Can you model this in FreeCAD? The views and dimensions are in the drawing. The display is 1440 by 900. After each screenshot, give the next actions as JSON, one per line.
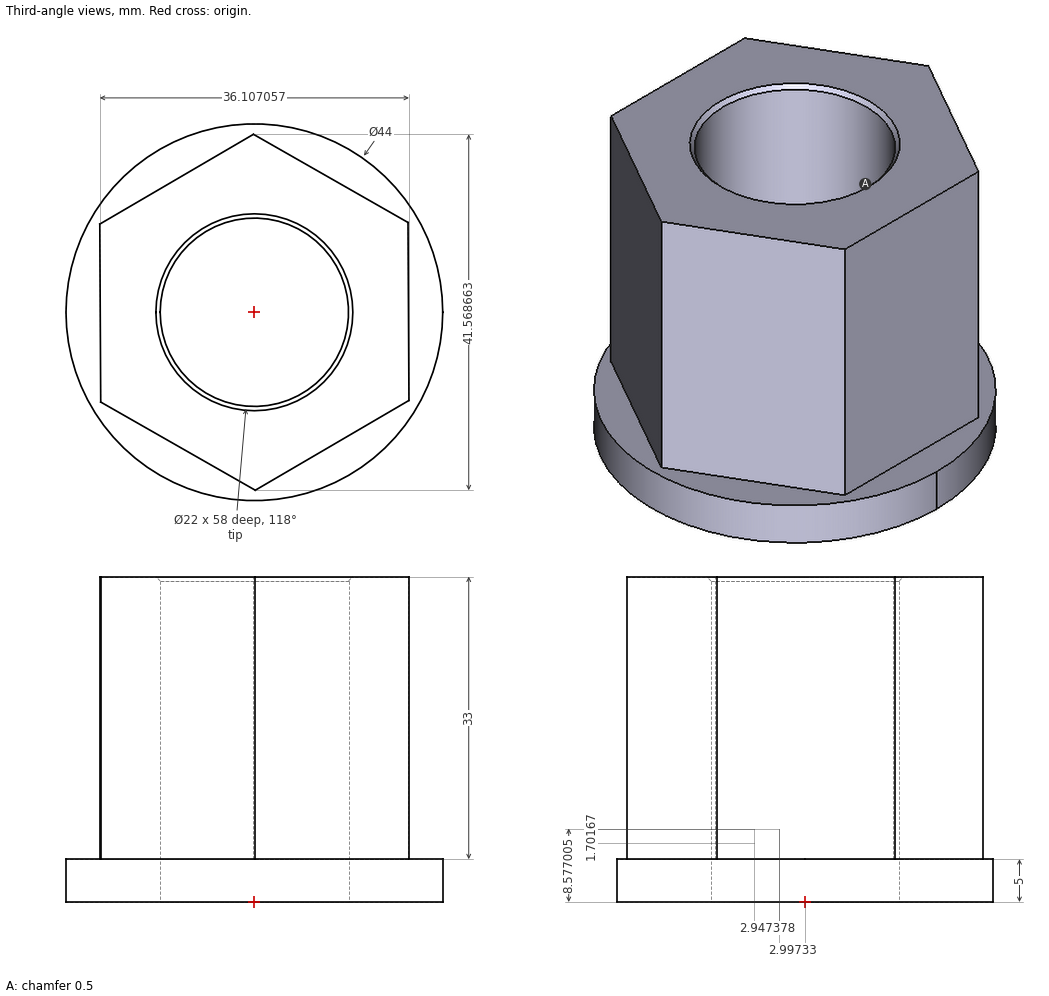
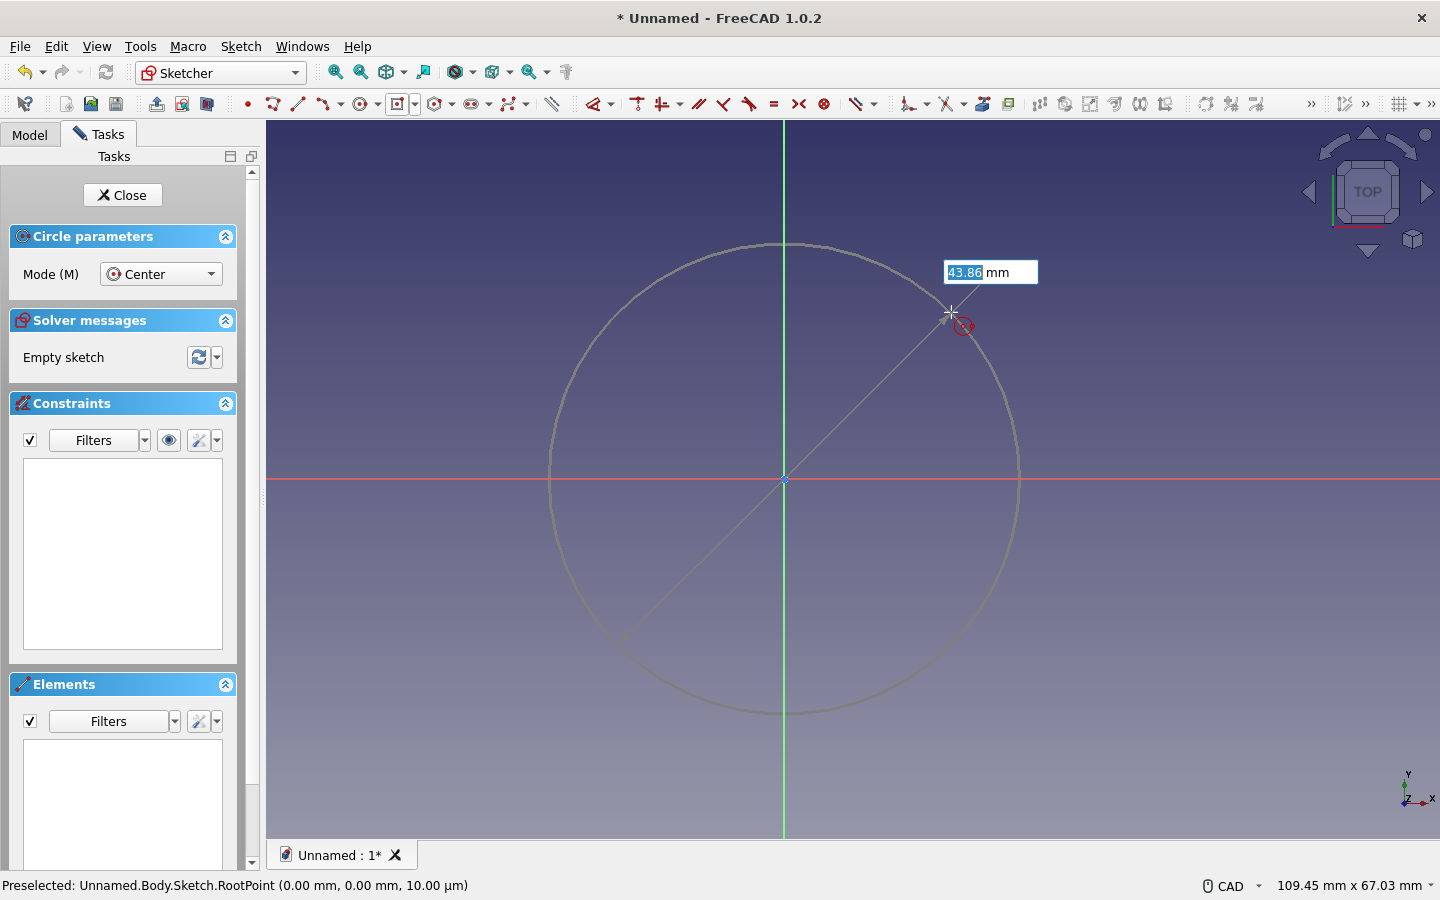
{"action": "type", "text": "44"}
{"action": "key", "text": "Return"}
{"action": "key", "text": "Escape"}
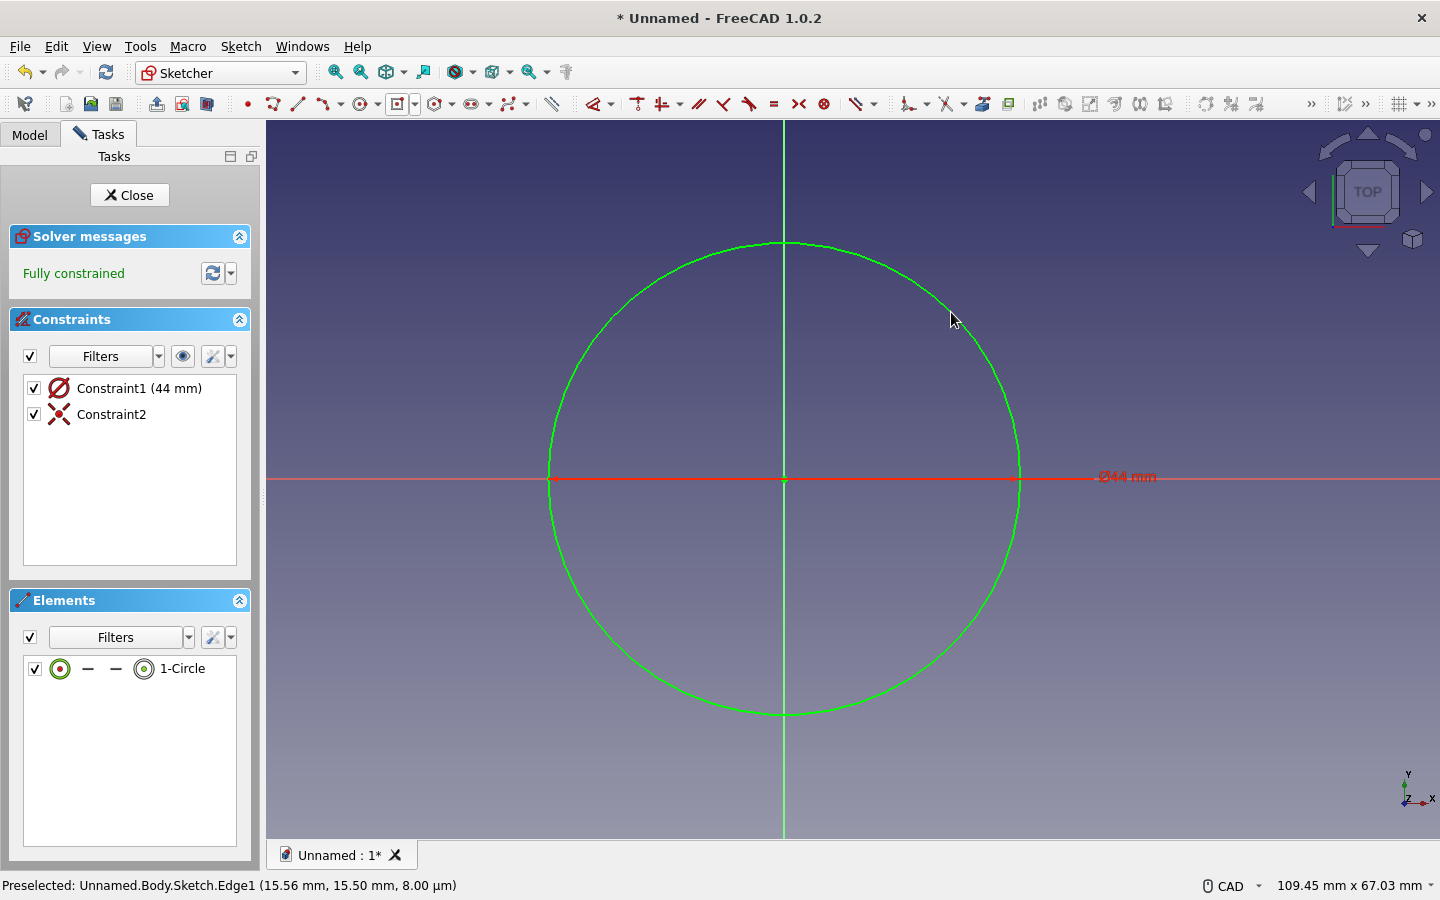
{"action": "left_click", "coordinate": [130, 195]}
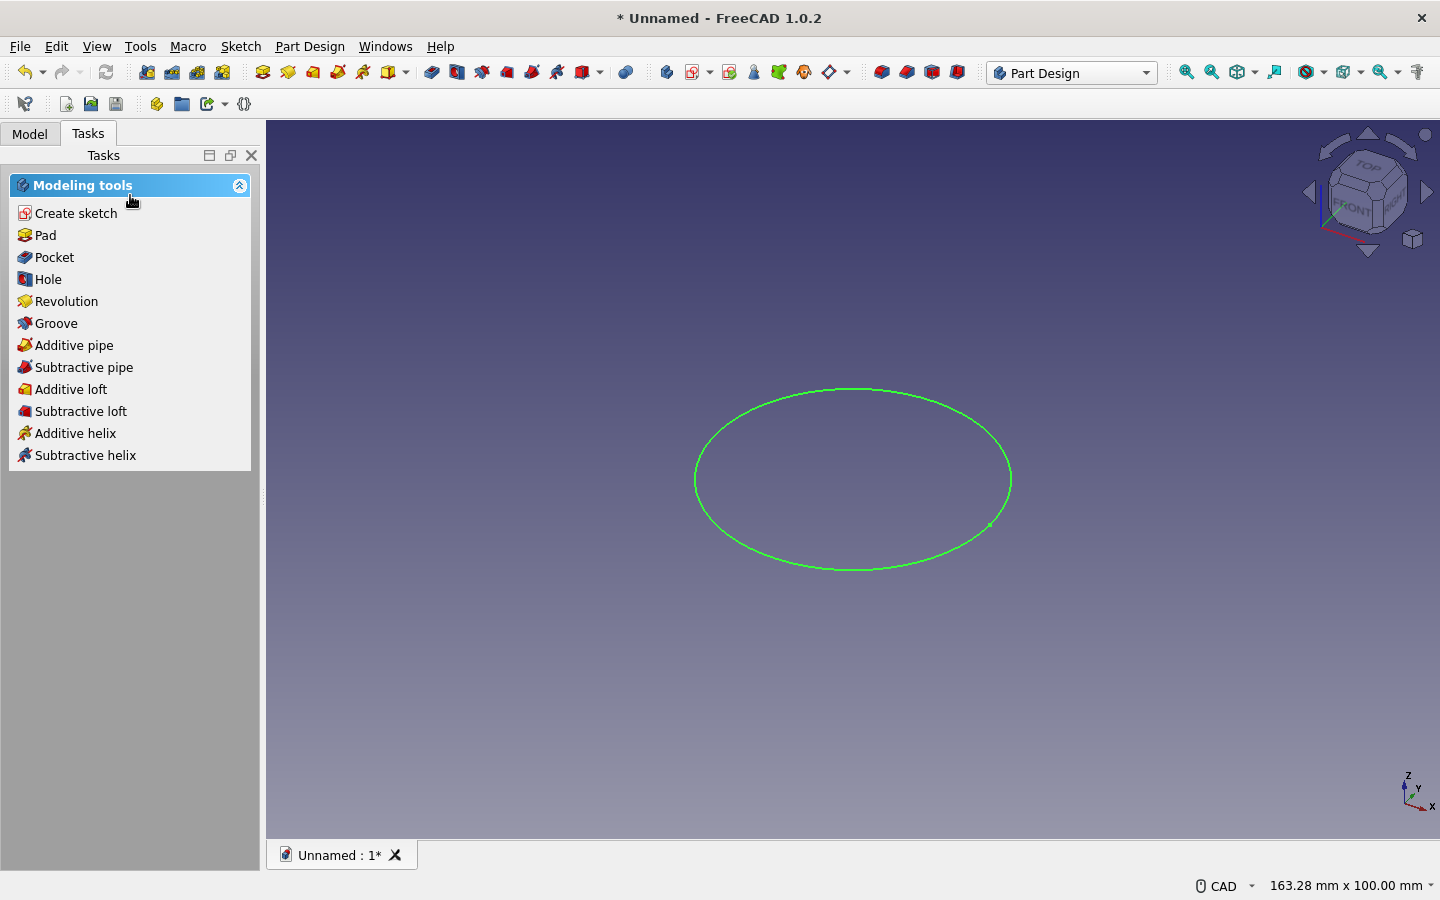
{"action": "left_click", "coordinate": [263, 72]}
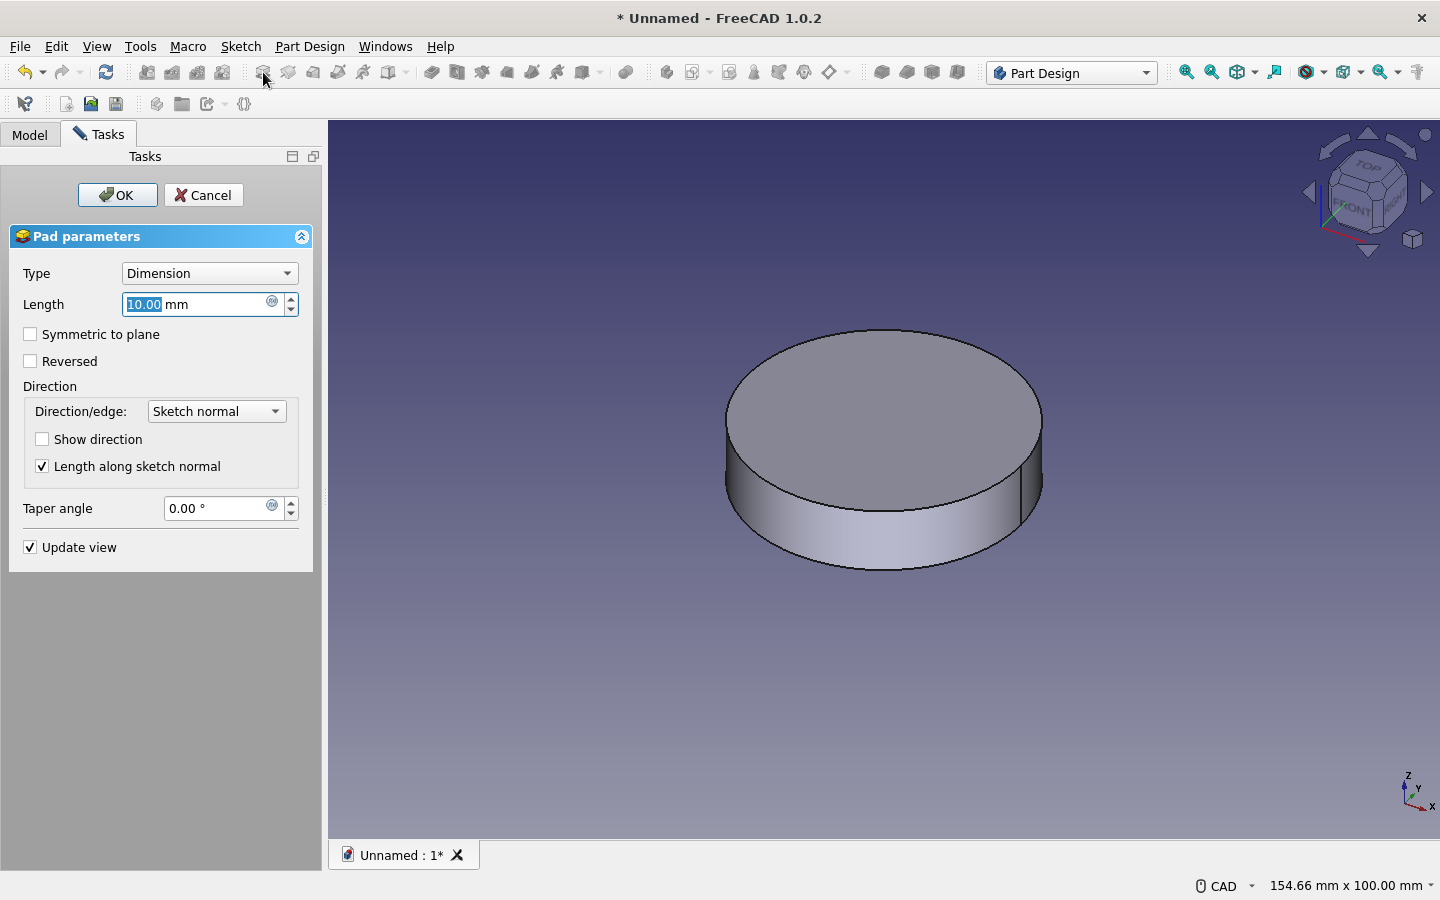
{"action": "type", "text": "5"}
{"action": "key", "text": "Tab"}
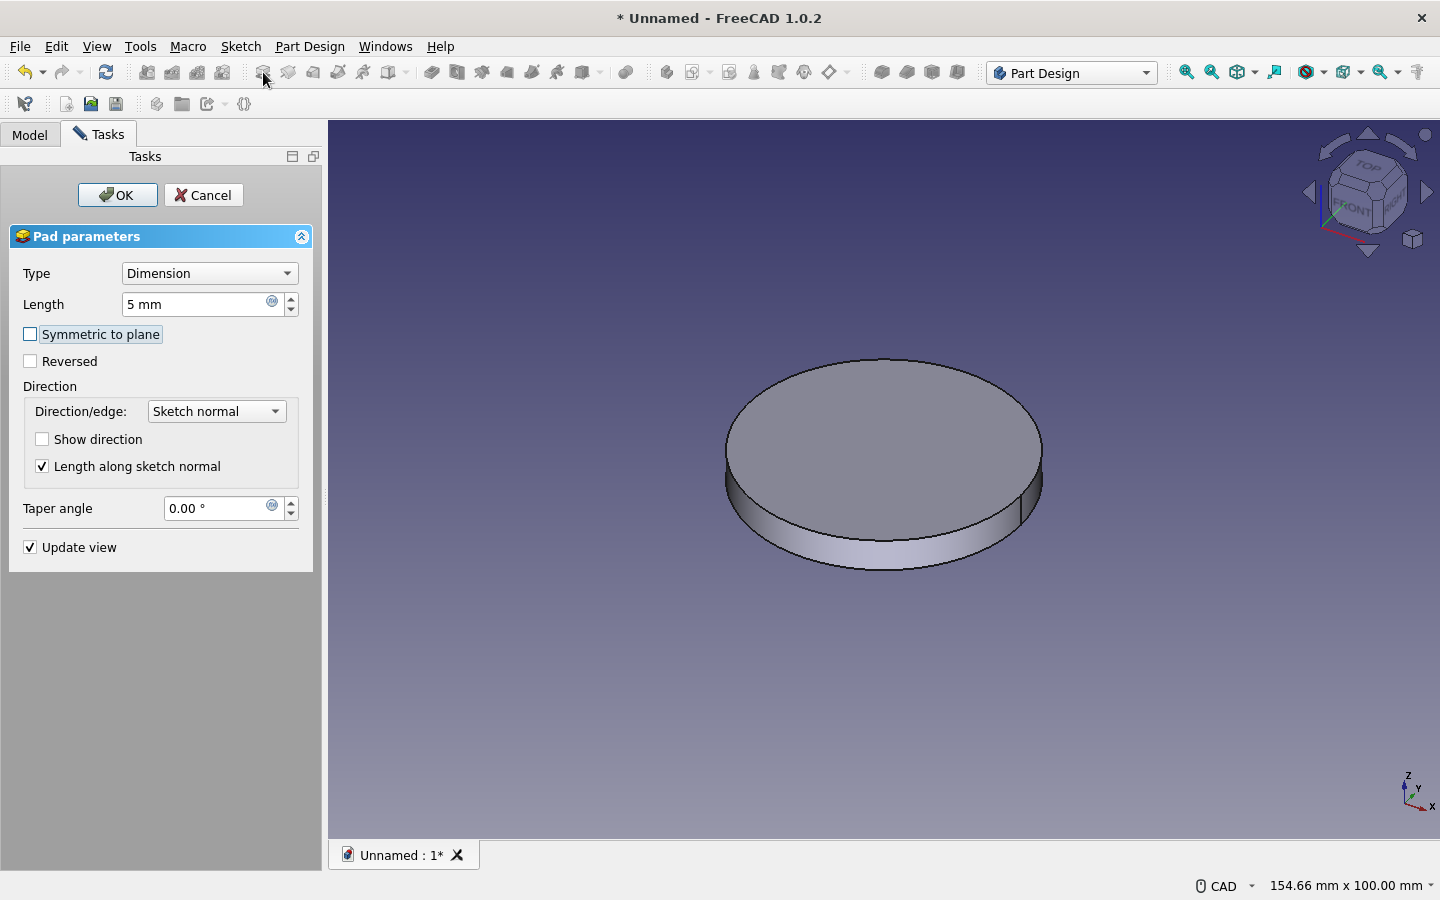
{"action": "left_click", "coordinate": [118, 195]}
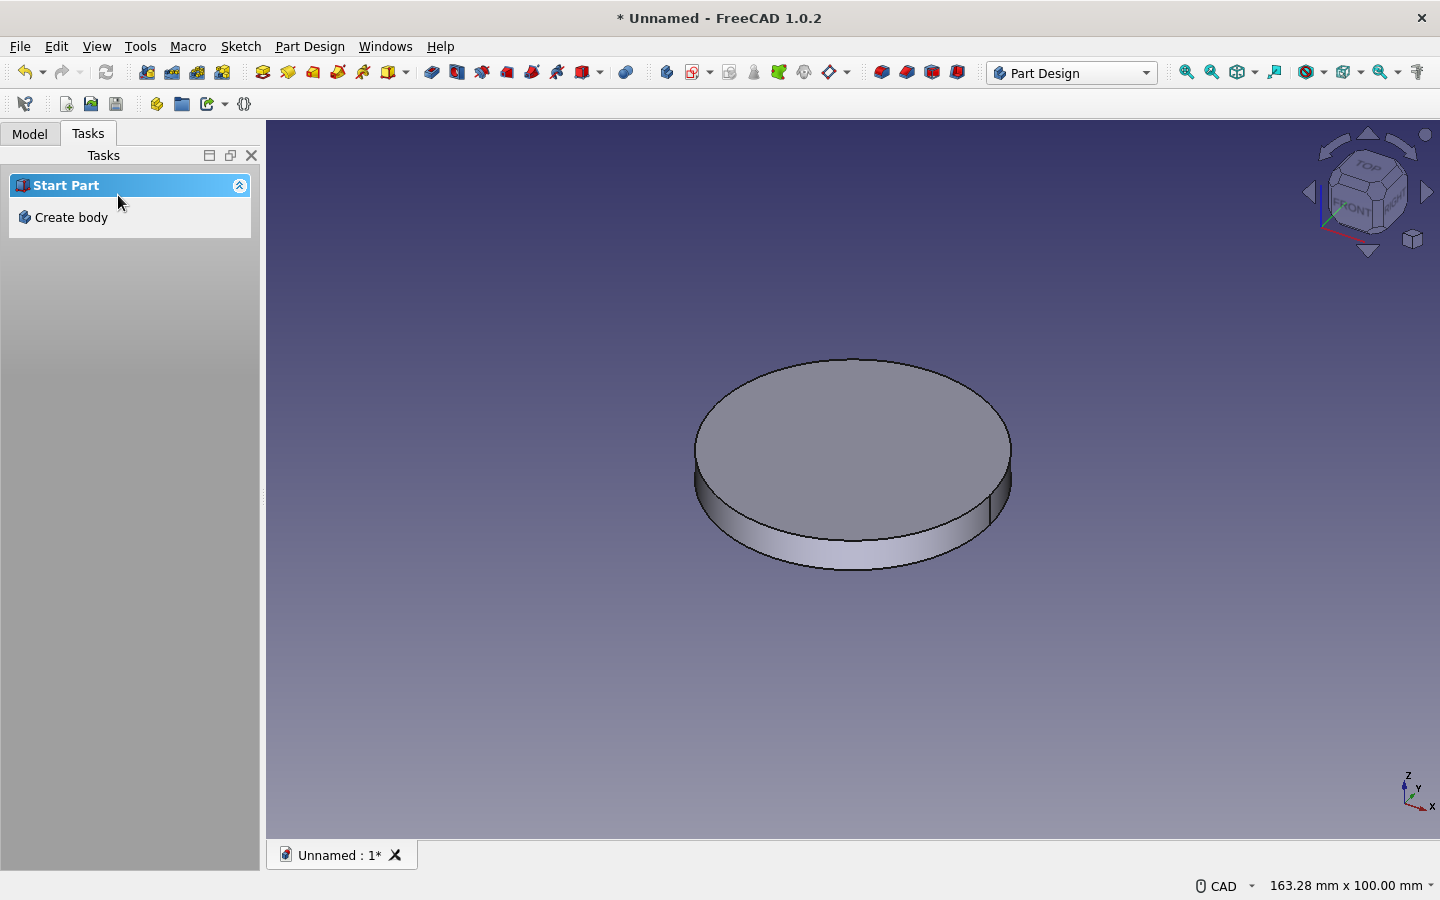
{"action": "key", "text": "v f"}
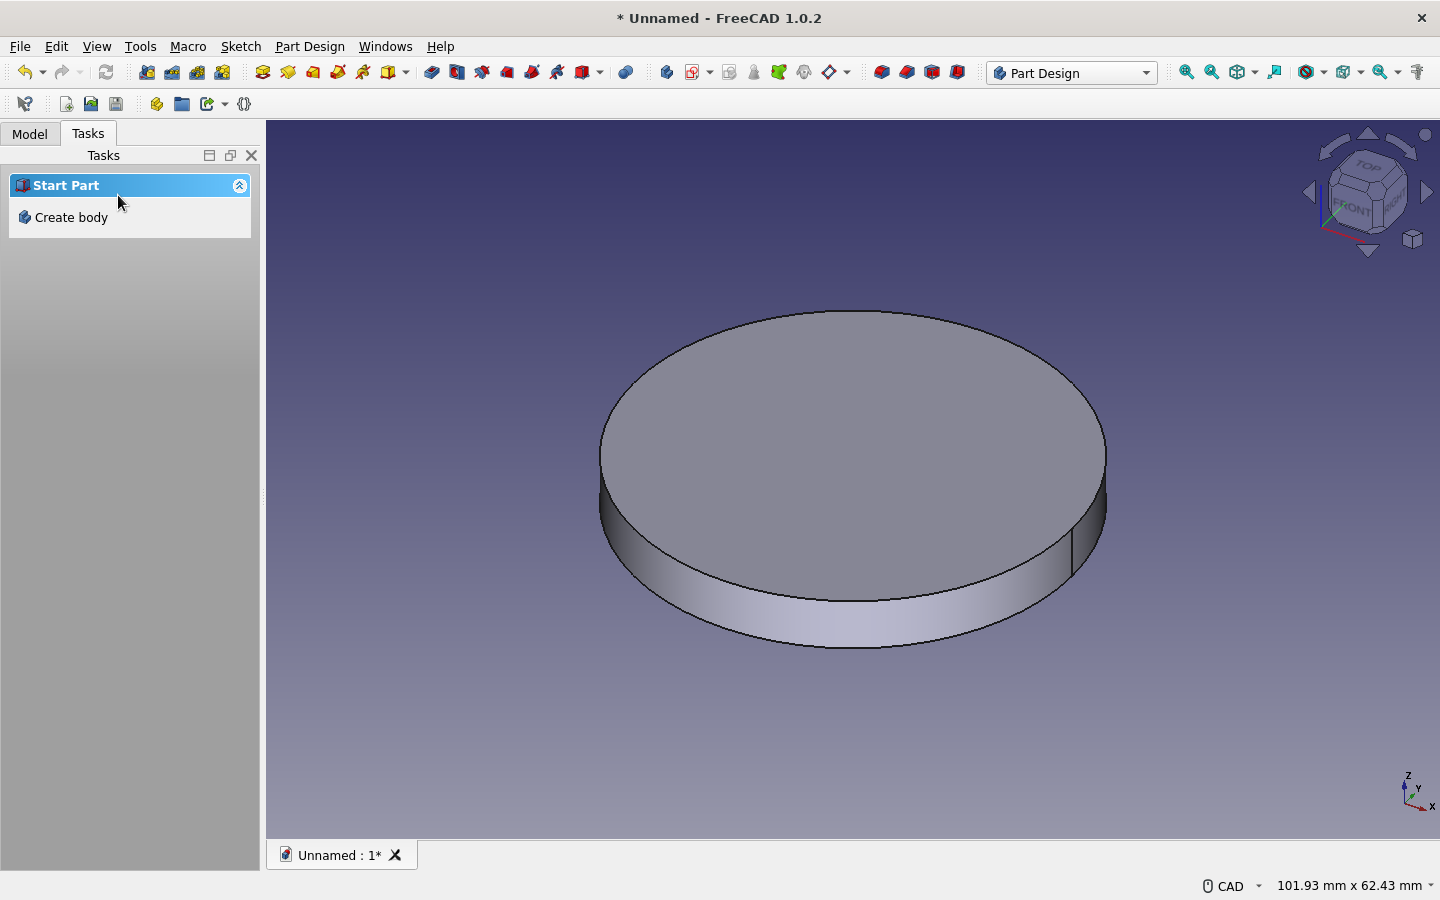
{"action": "left_click", "coordinate": [853, 455]}